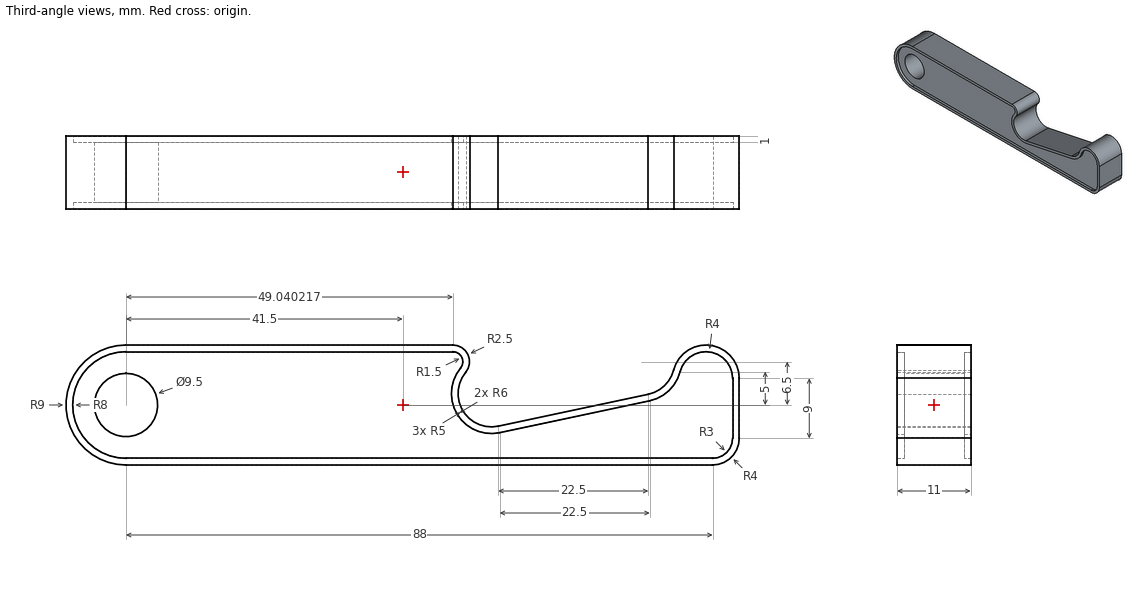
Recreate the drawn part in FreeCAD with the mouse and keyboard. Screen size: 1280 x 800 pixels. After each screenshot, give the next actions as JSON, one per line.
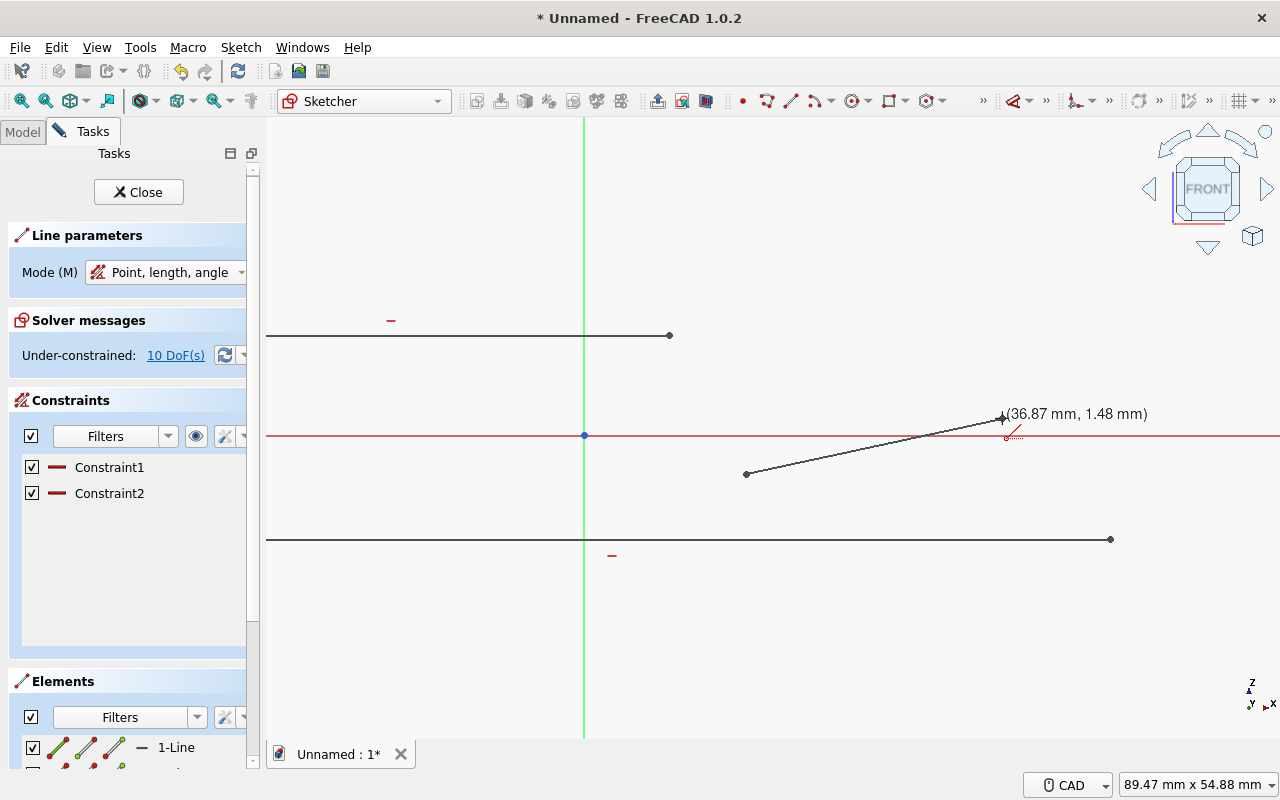
{"action": "scroll", "coordinate": [851, 418], "scroll_direction": "down", "scroll_amount": 3}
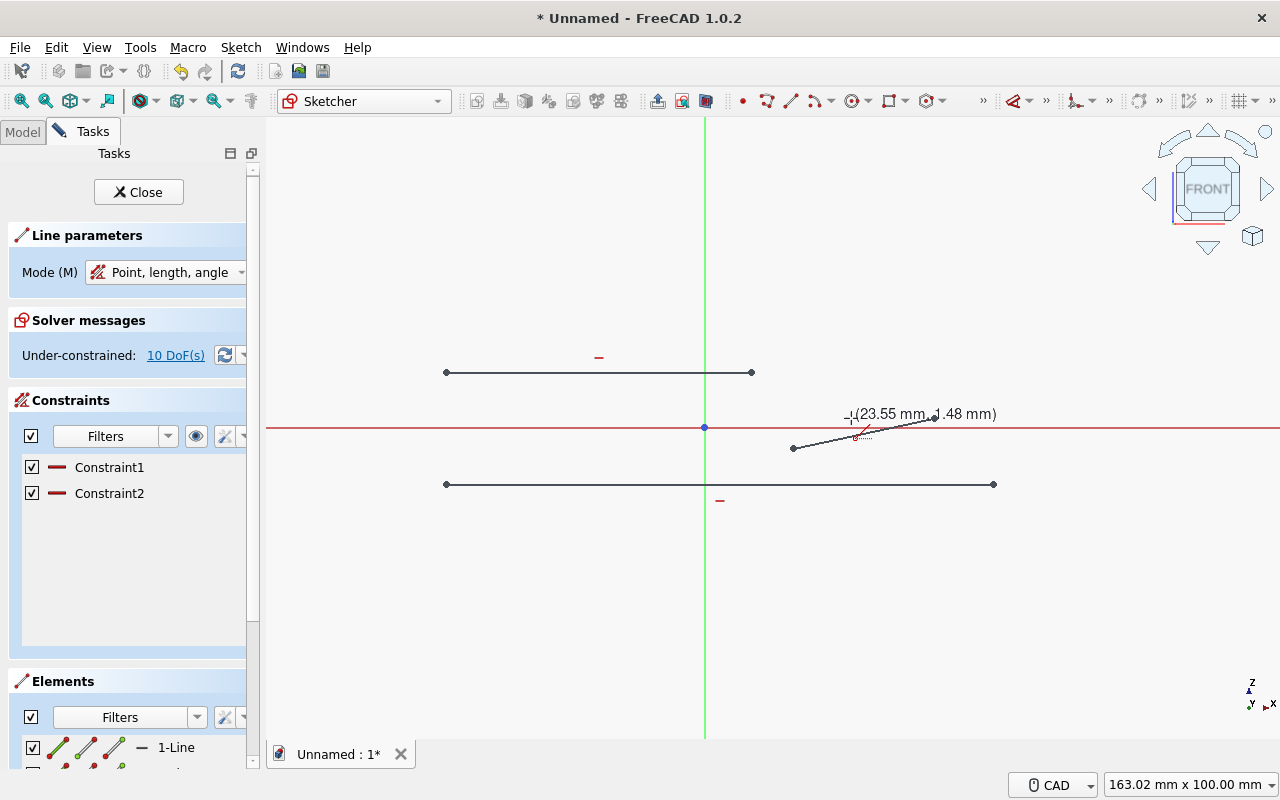
{"action": "left_click", "coordinate": [1019, 403]}
{"action": "left_click", "coordinate": [1019, 459]}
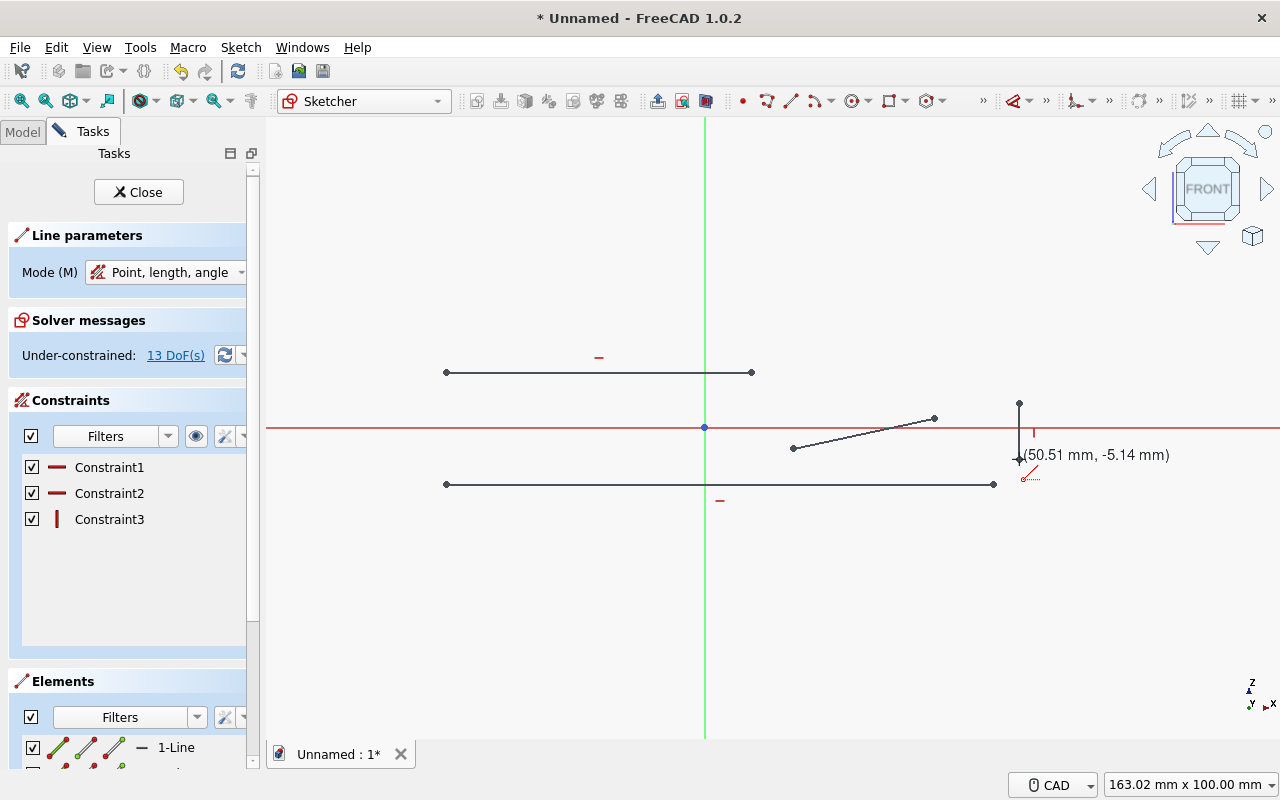
{"action": "left_click", "coordinate": [834, 102]}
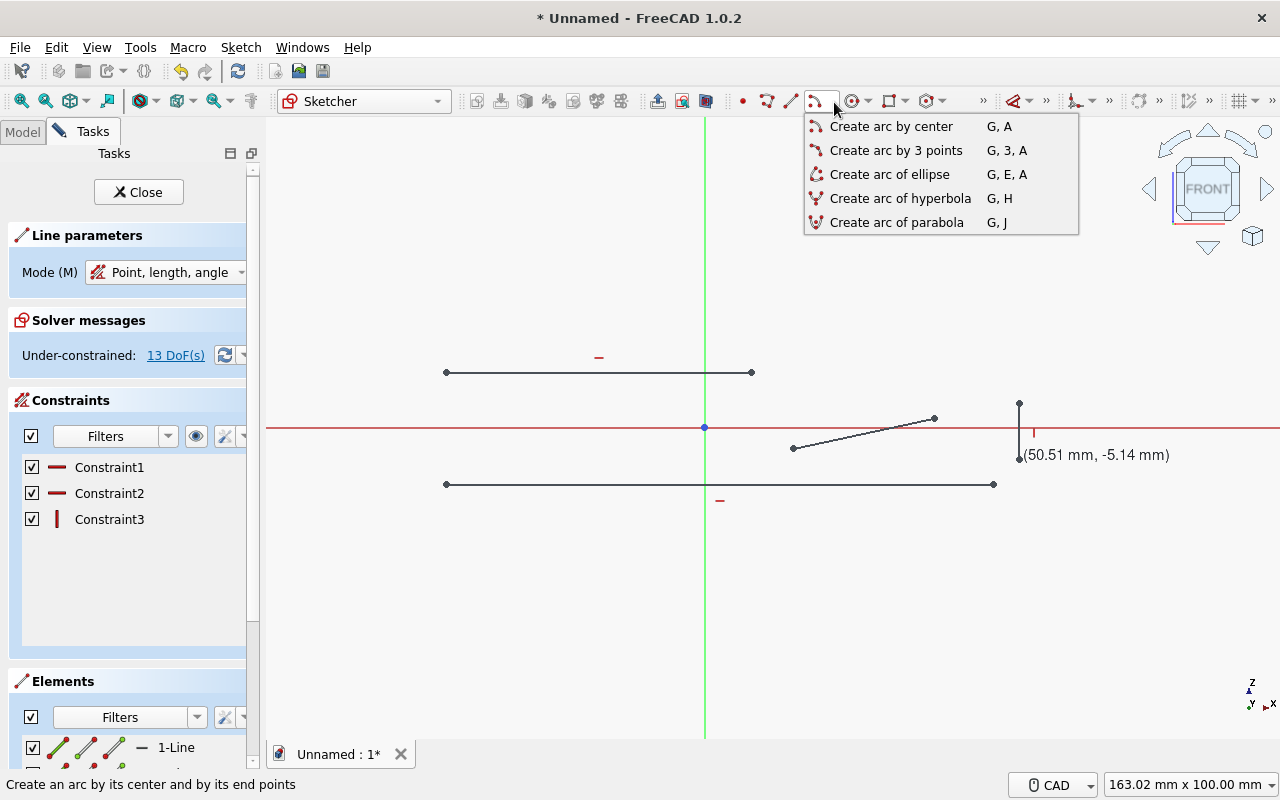
{"action": "left_click", "coordinate": [942, 150]}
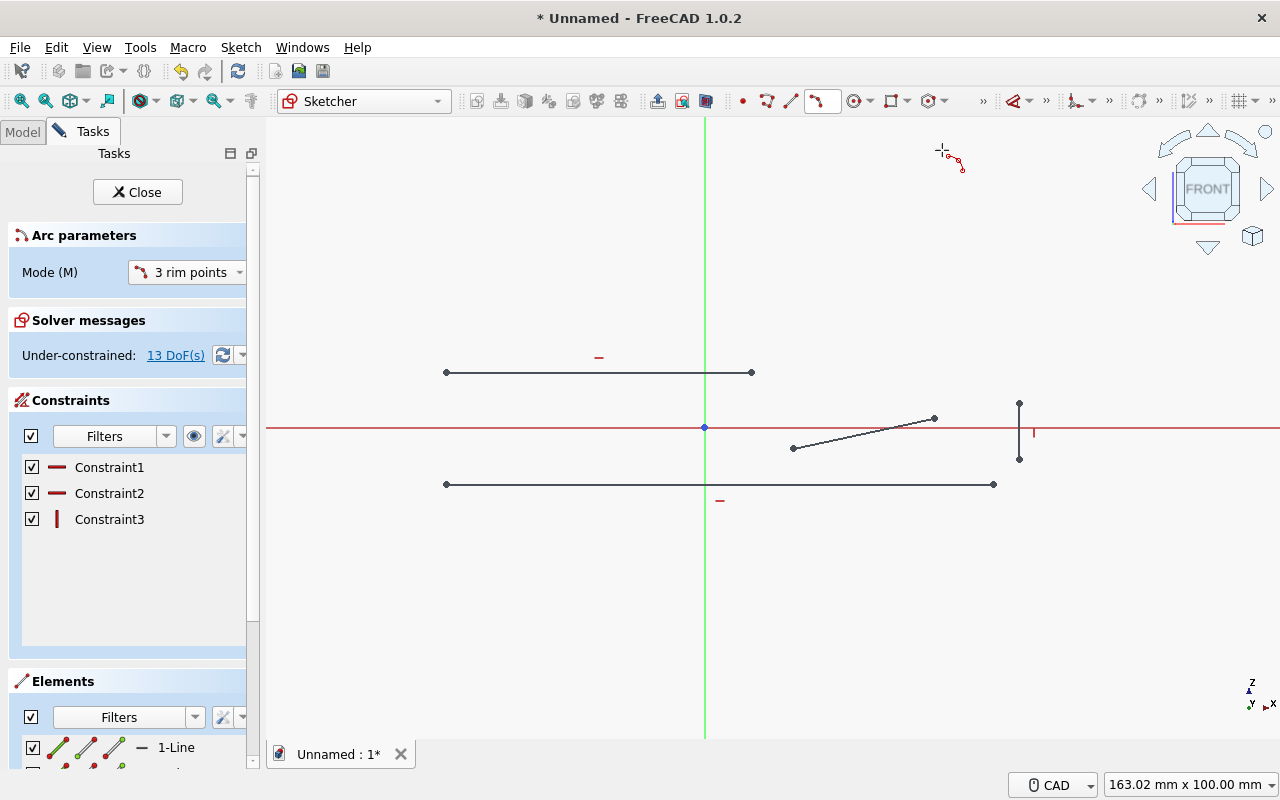
{"action": "left_click", "coordinate": [447, 485]}
{"action": "left_click", "coordinate": [447, 373]}
{"action": "left_click", "coordinate": [393, 411]}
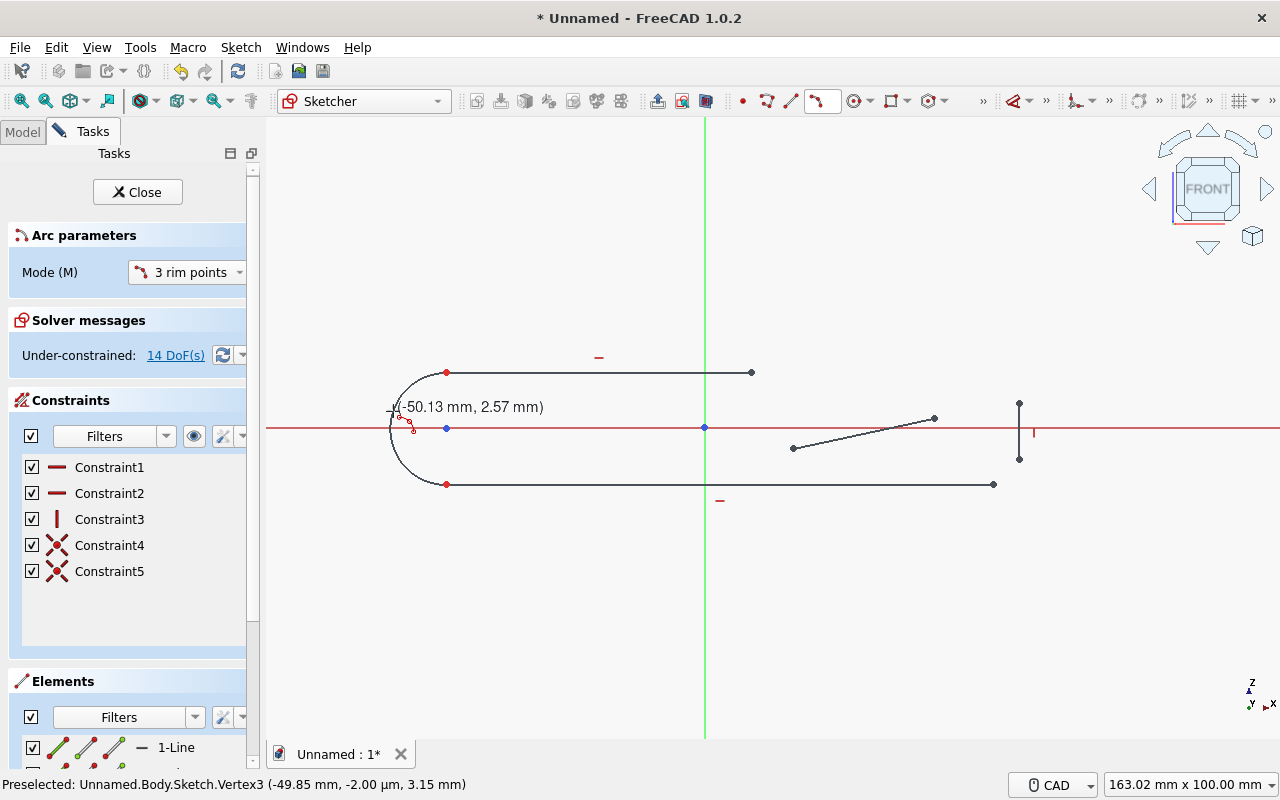
{"action": "left_click", "coordinate": [752, 373]}
{"action": "left_click", "coordinate": [764, 397]}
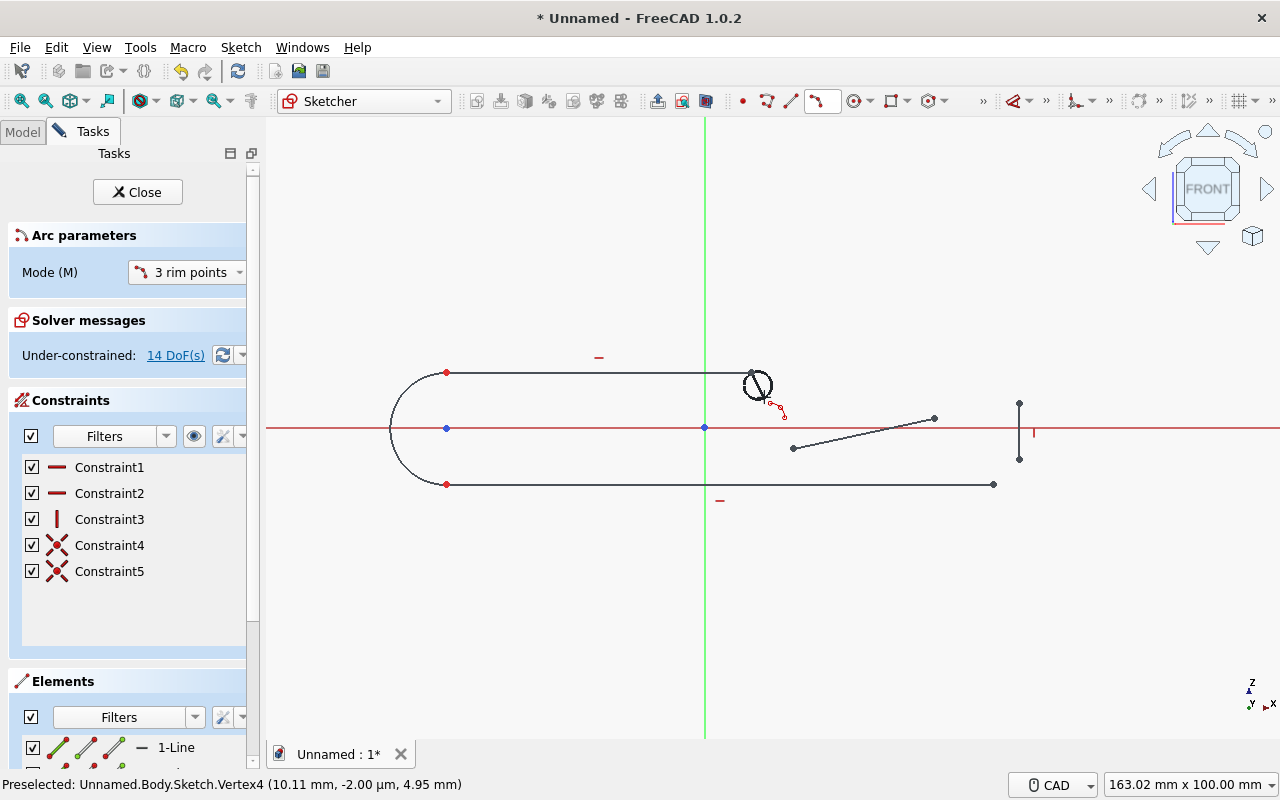
{"action": "scroll", "coordinate": [766, 381], "scroll_direction": "up", "scroll_amount": 3}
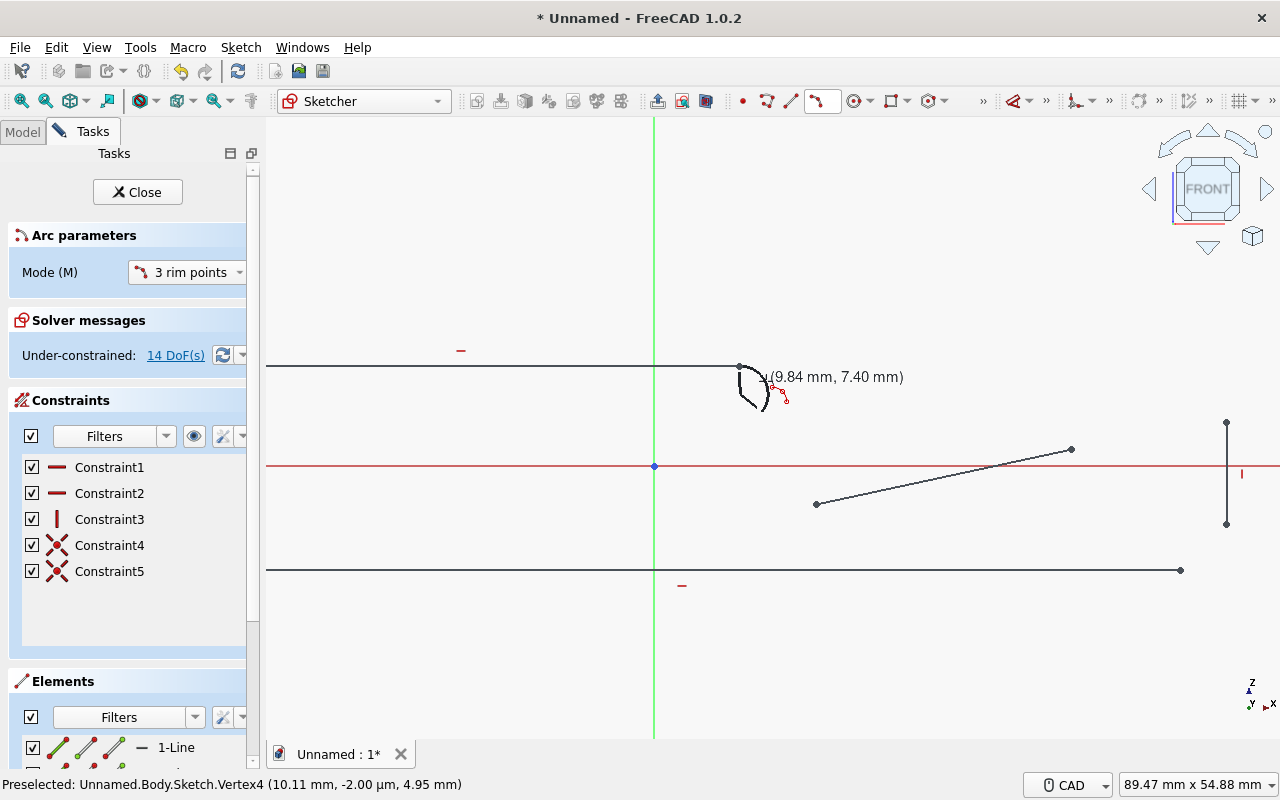
{"action": "left_click", "coordinate": [765, 381]}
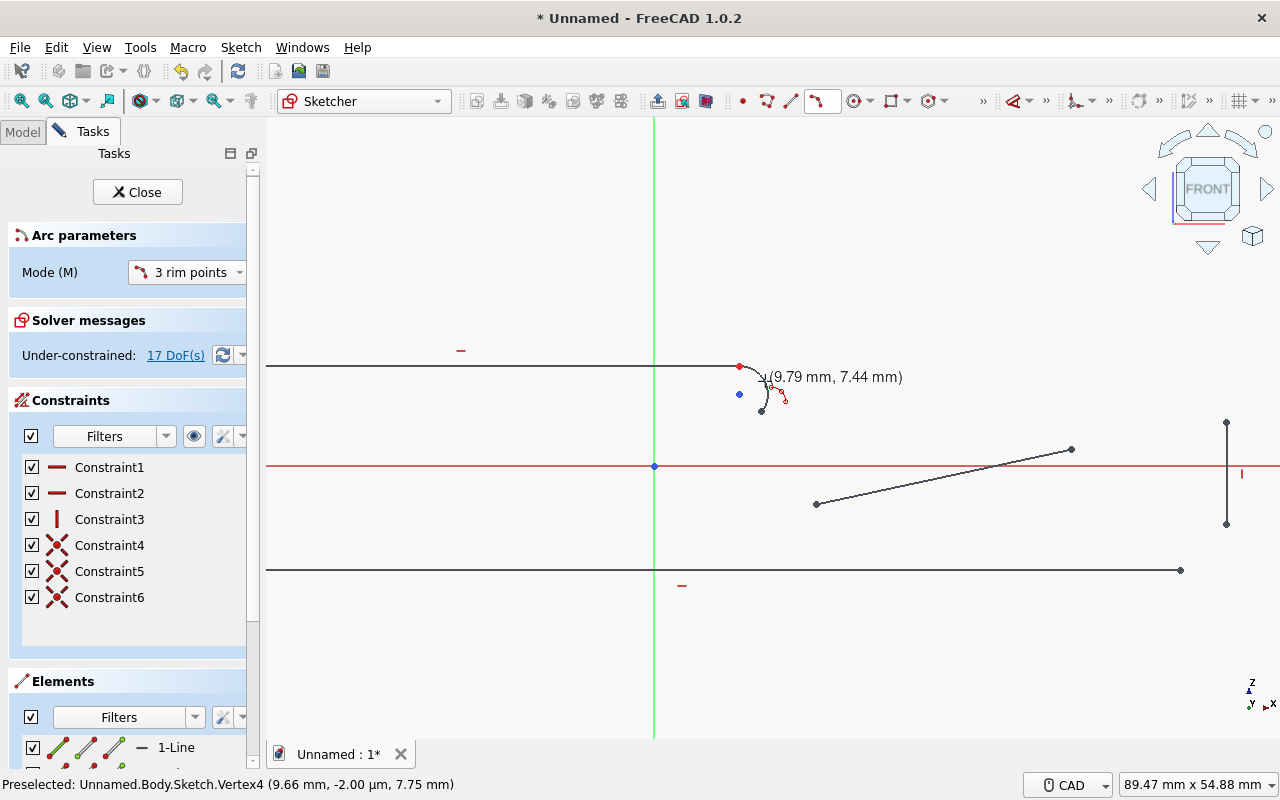
{"action": "left_click", "coordinate": [762, 412]}
{"action": "left_click", "coordinate": [816, 505]}
{"action": "left_click", "coordinate": [776, 496]}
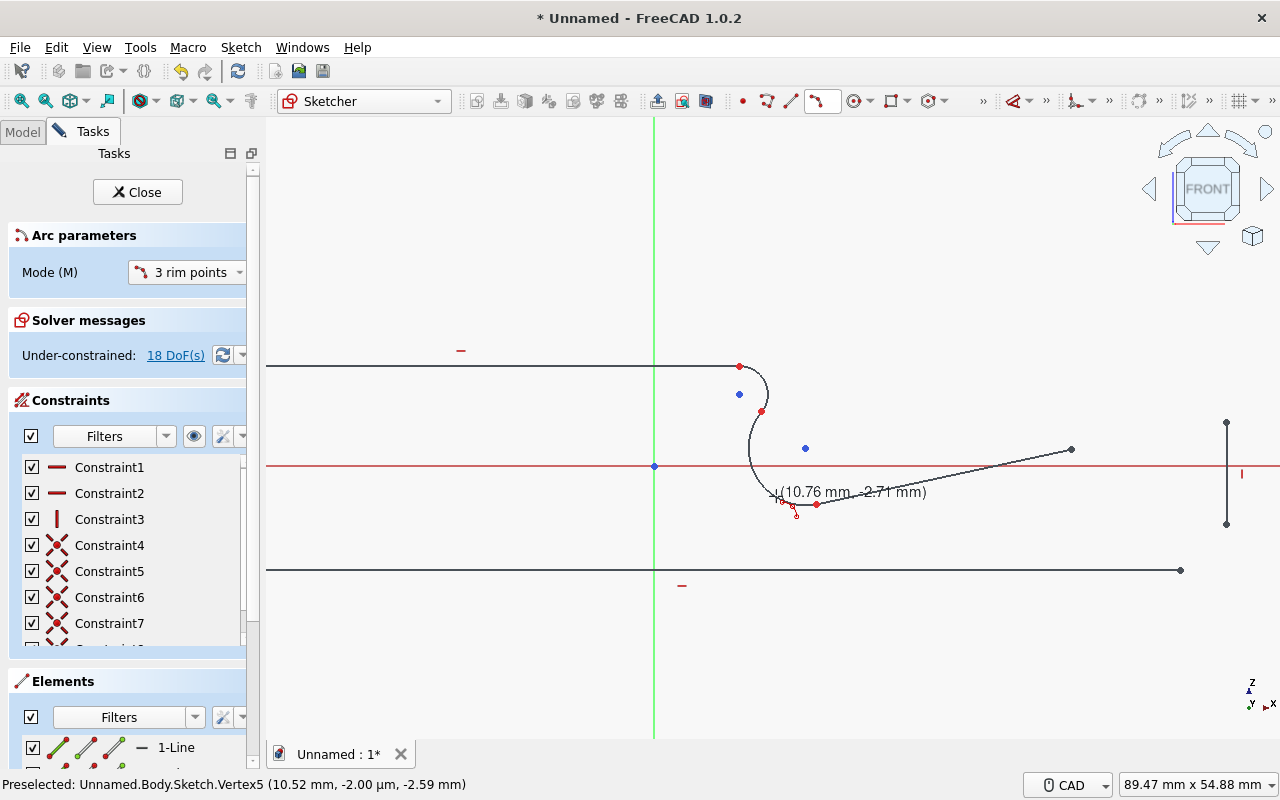
{"action": "left_click", "coordinate": [1072, 449]}
{"action": "left_click", "coordinate": [1115, 407]}